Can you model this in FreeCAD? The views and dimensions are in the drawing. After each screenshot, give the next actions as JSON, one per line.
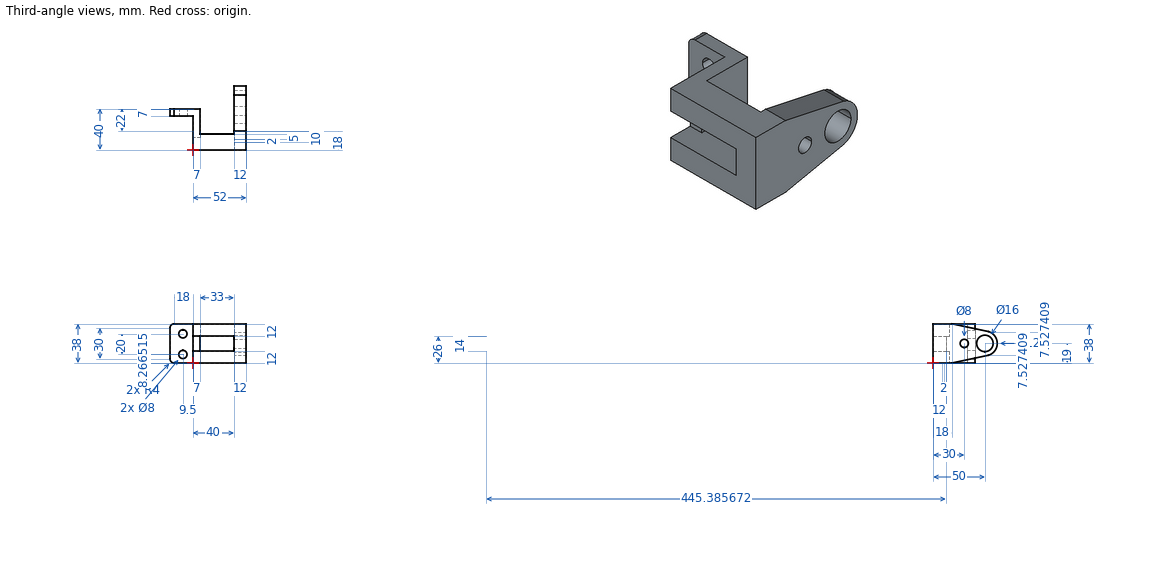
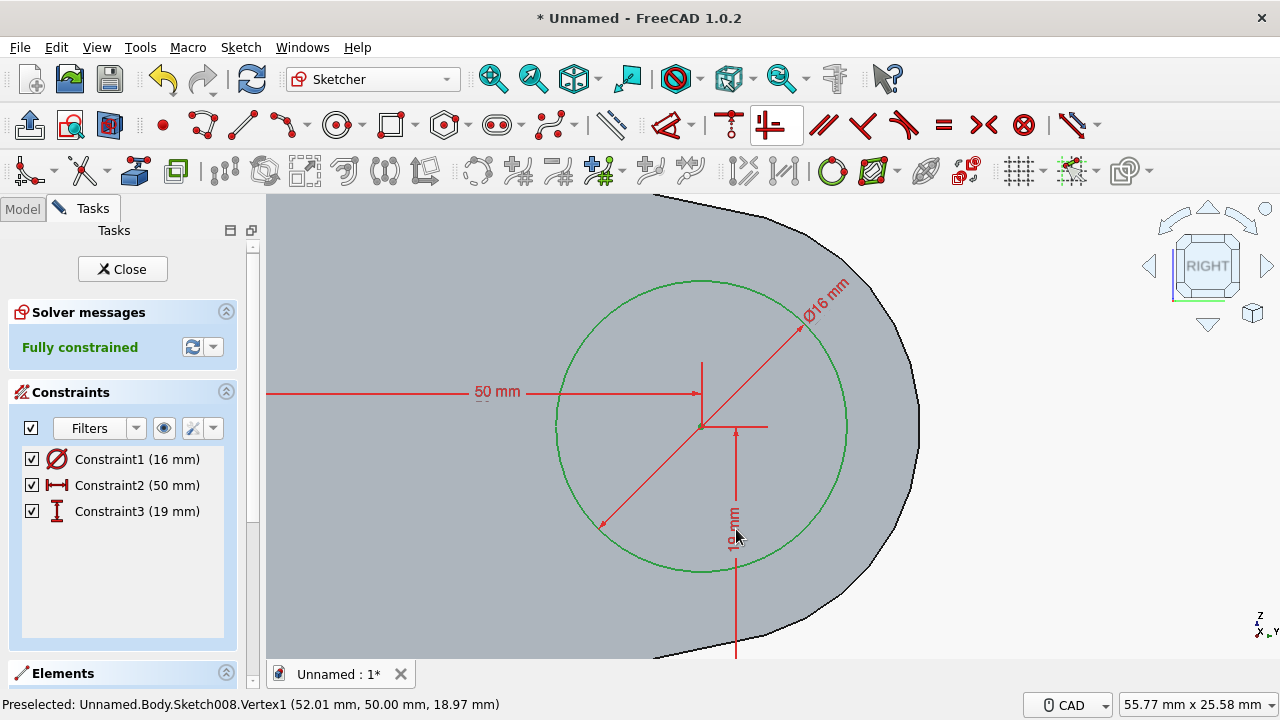
{"action": "left_click", "coordinate": [123, 269]}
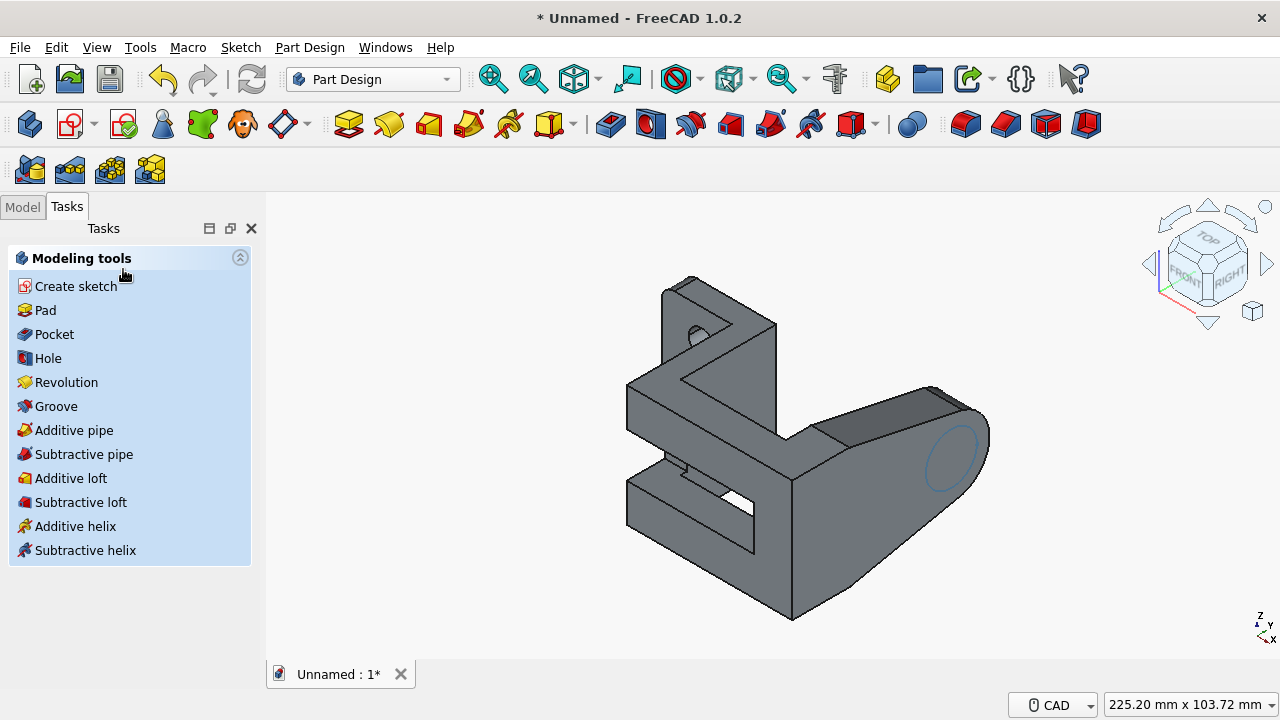
{"action": "left_click", "coordinate": [612, 124]}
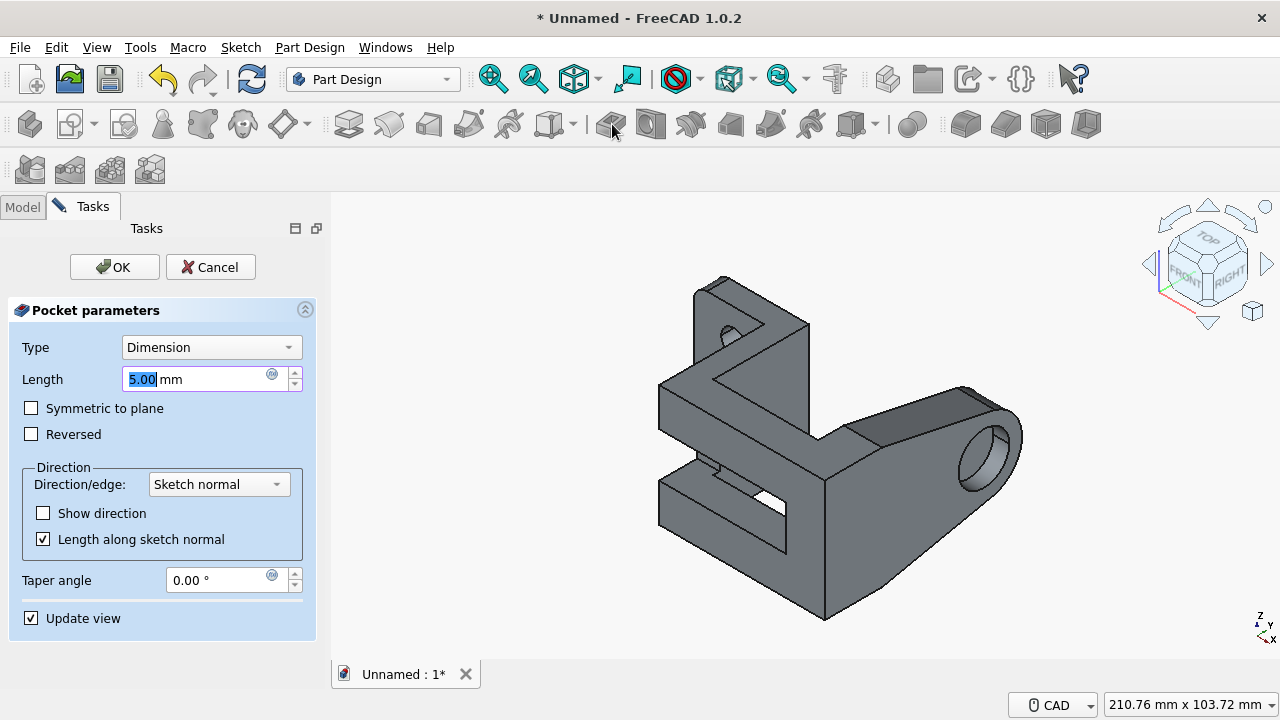
{"action": "type", "text": "12"}
{"action": "key", "text": "Tab"}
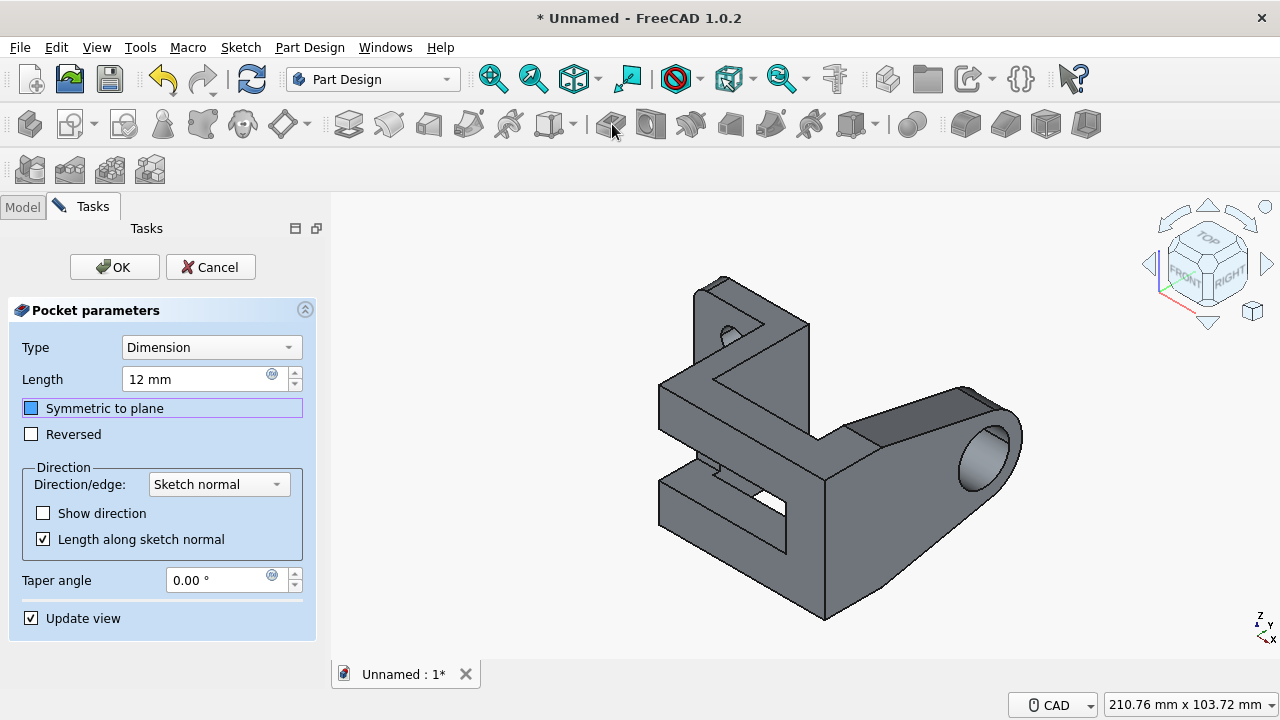
{"action": "left_click", "coordinate": [115, 267]}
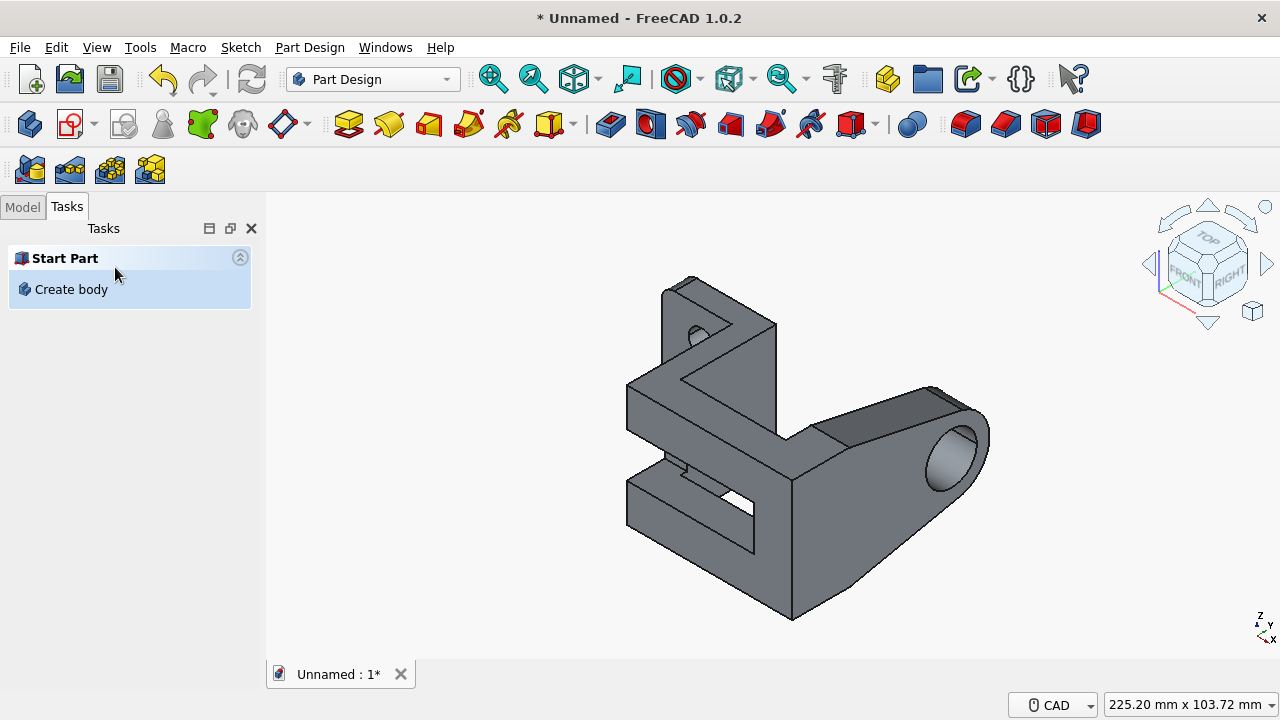
{"action": "left_click", "coordinate": [863, 509]}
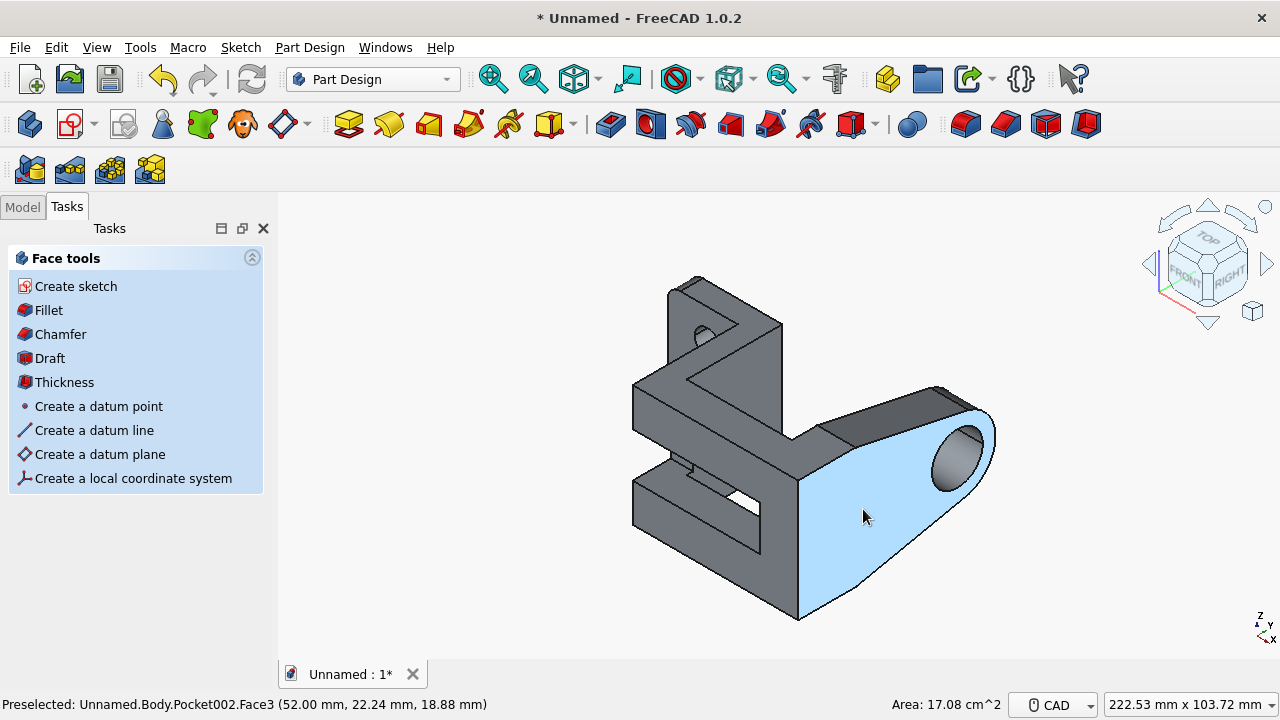
{"action": "left_click", "coordinate": [70, 124]}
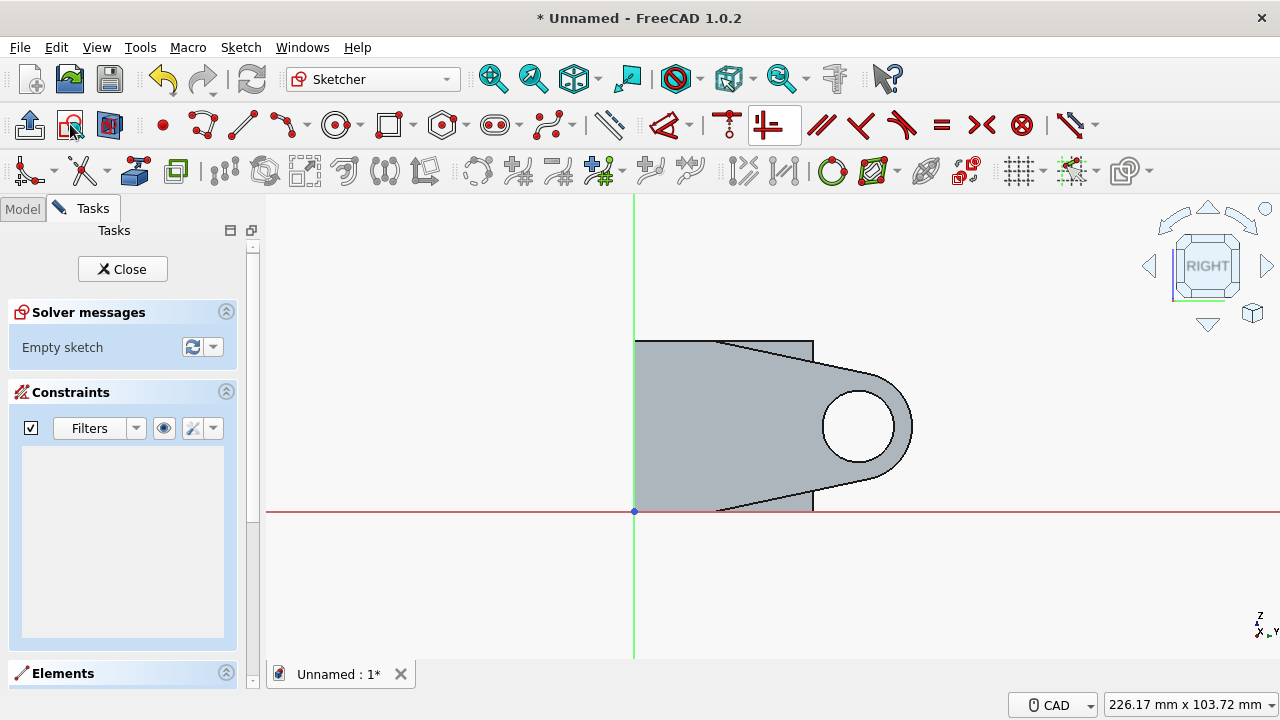
{"action": "scroll", "coordinate": [779, 426], "scroll_direction": "up", "scroll_amount": 10}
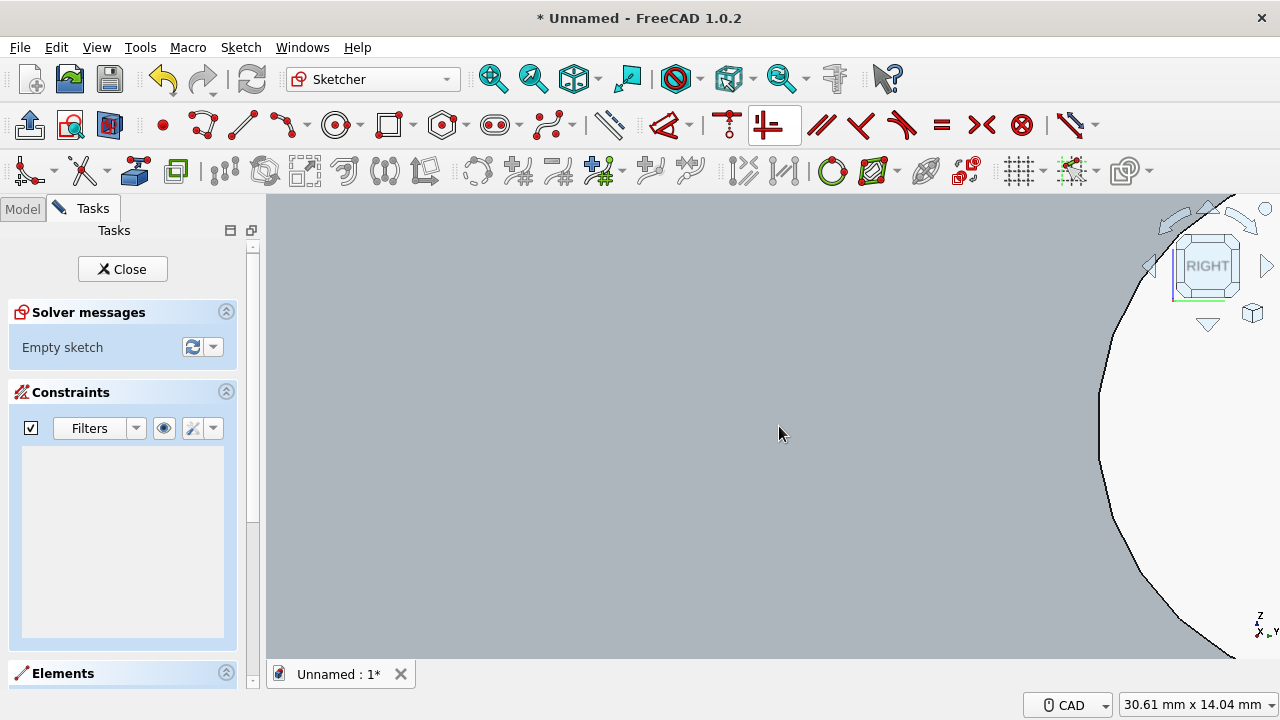
{"action": "left_click", "coordinate": [336, 126]}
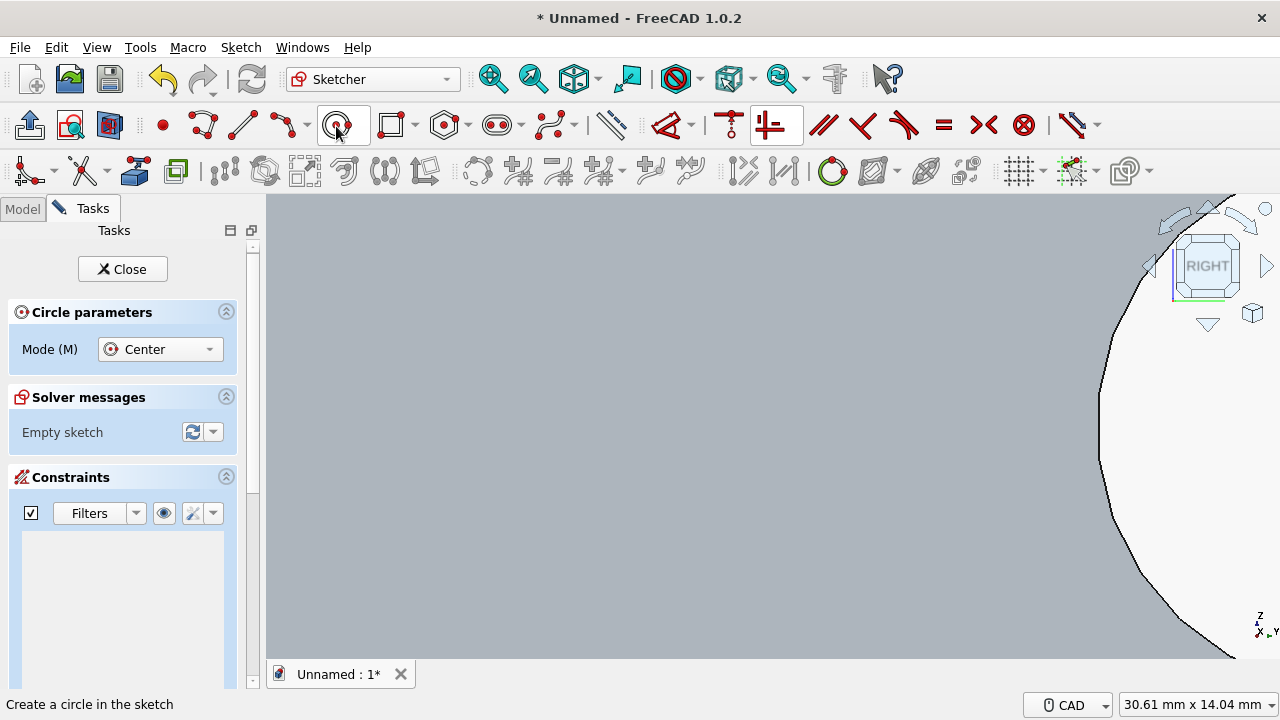
{"action": "left_click", "coordinate": [699, 426]}
{"action": "left_click", "coordinate": [793, 333]}
{"action": "key", "text": "Escape"}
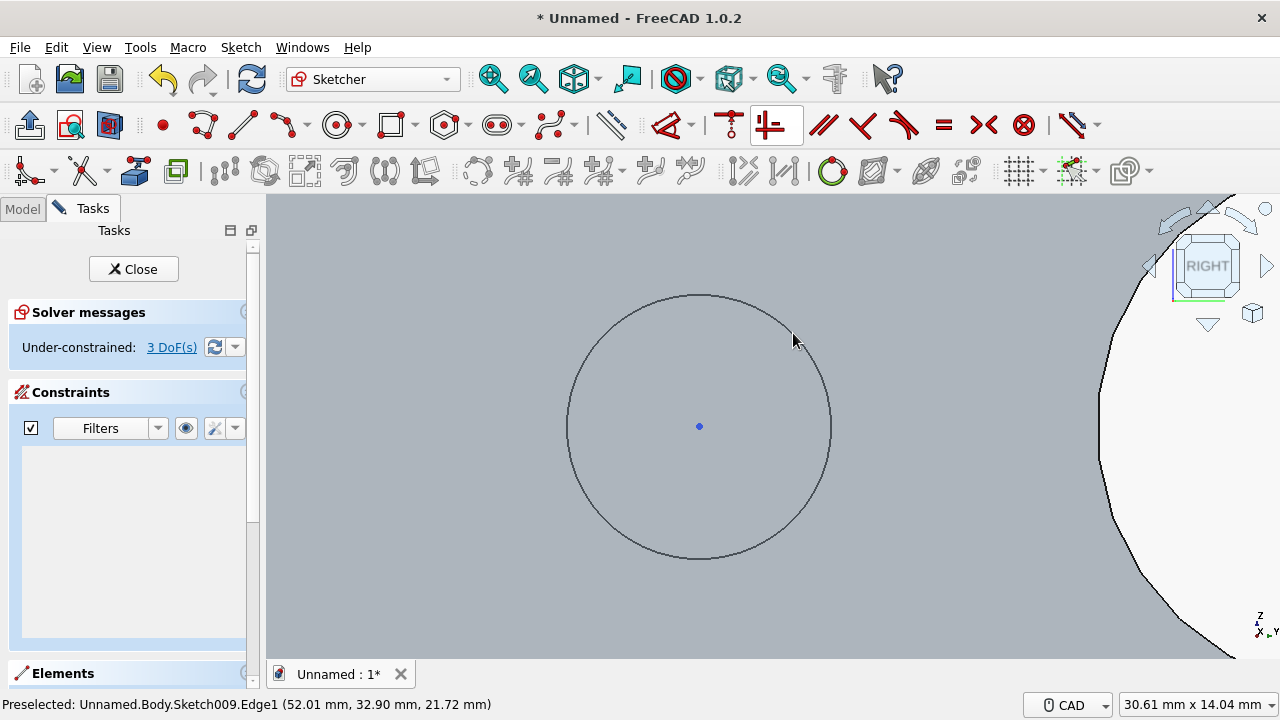
{"action": "left_click", "coordinate": [666, 126]}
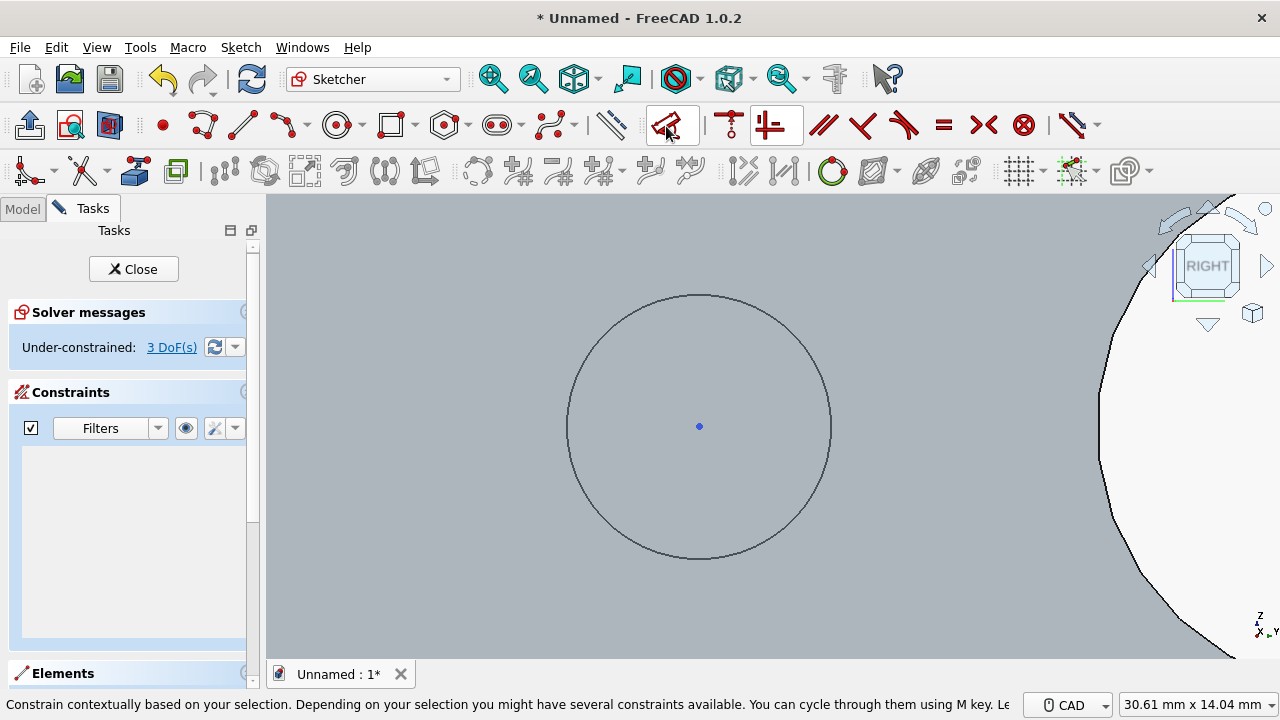
{"action": "left_click", "coordinate": [792, 333]}
{"action": "left_click", "coordinate": [815, 310]}